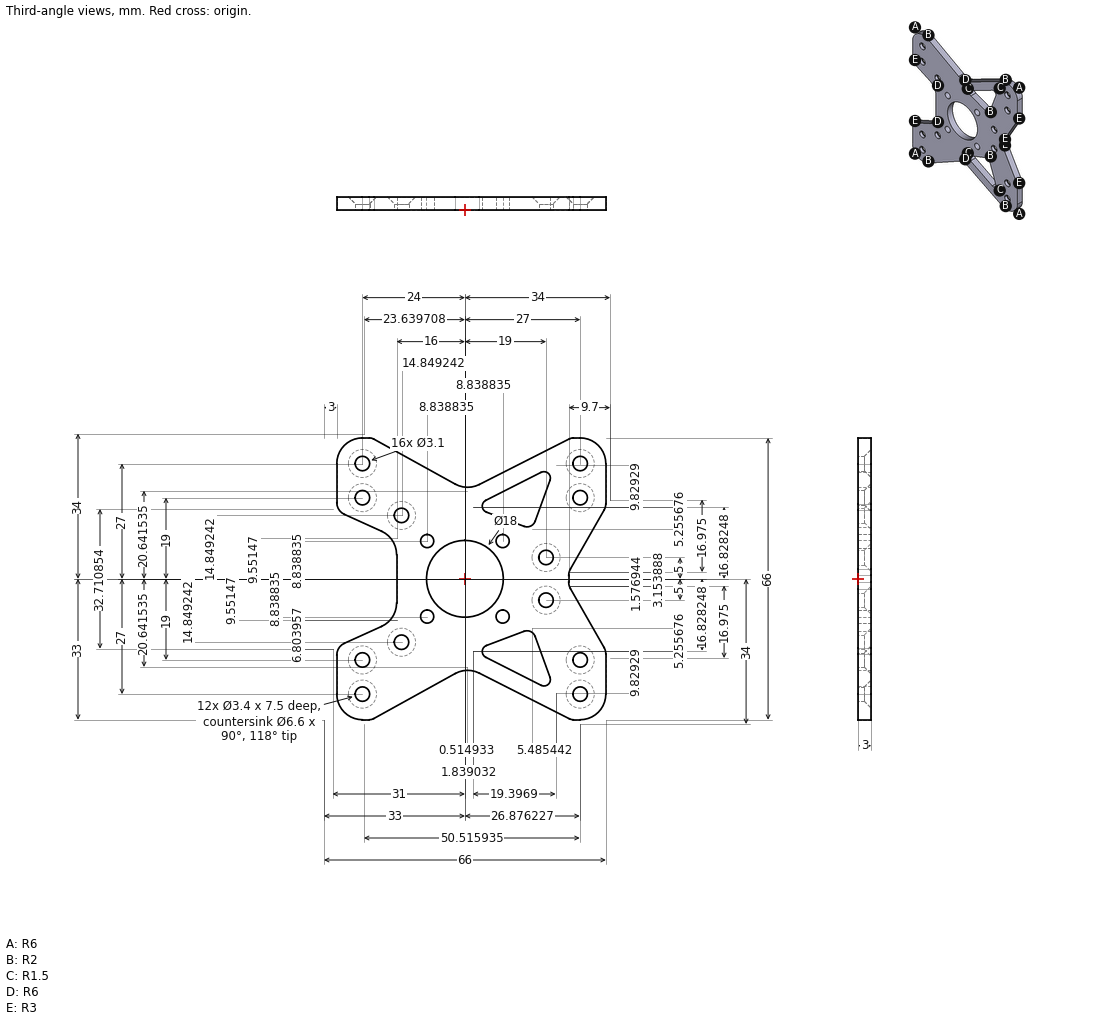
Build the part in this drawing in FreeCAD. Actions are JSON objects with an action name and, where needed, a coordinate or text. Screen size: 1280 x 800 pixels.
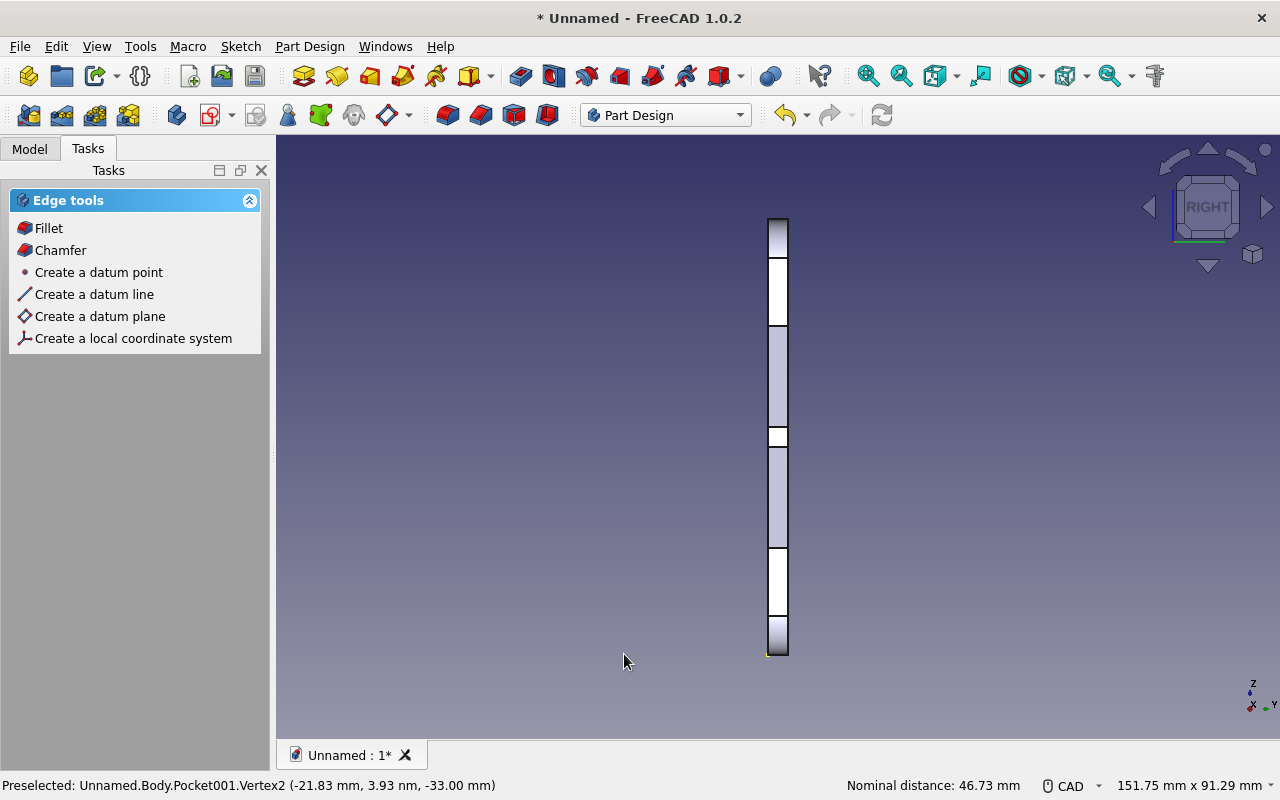
{"action": "scroll", "coordinate": [778, 654], "scroll_direction": "up", "scroll_amount": 4}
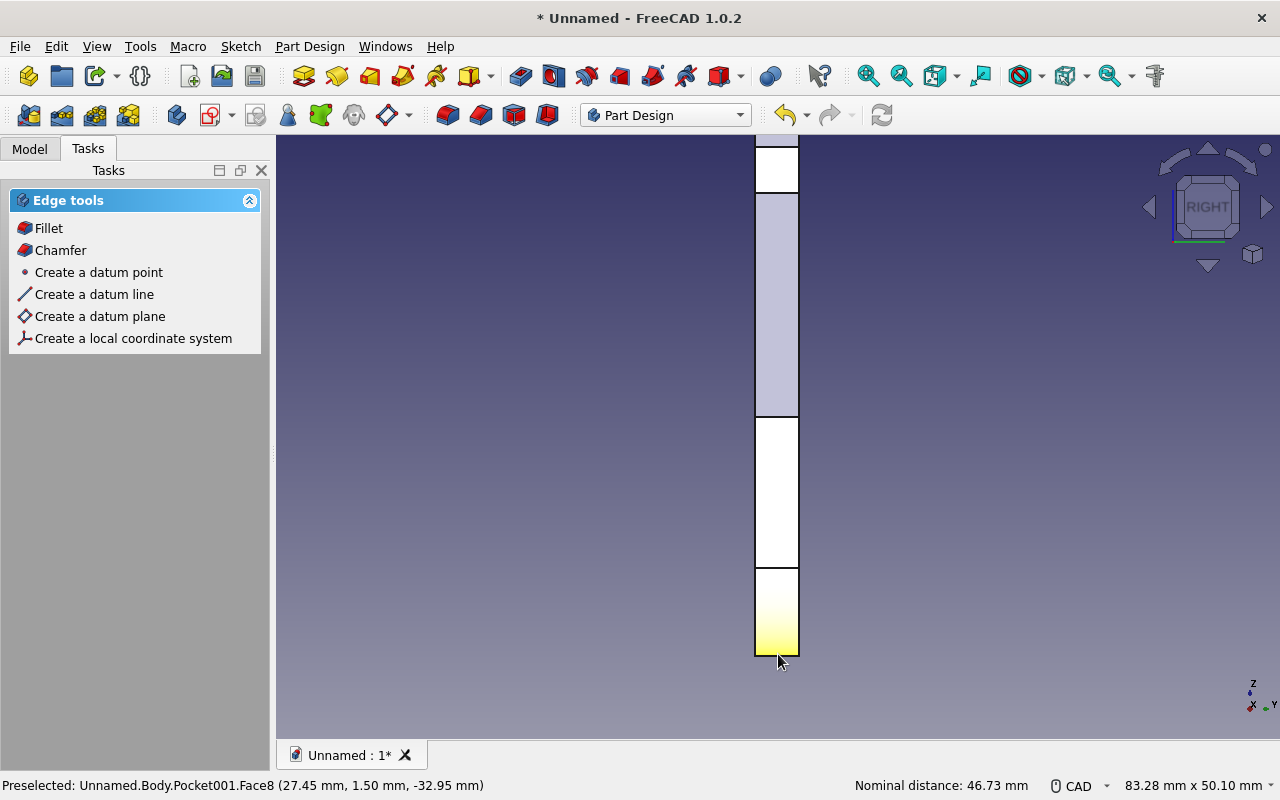
{"action": "key", "text": "v f"}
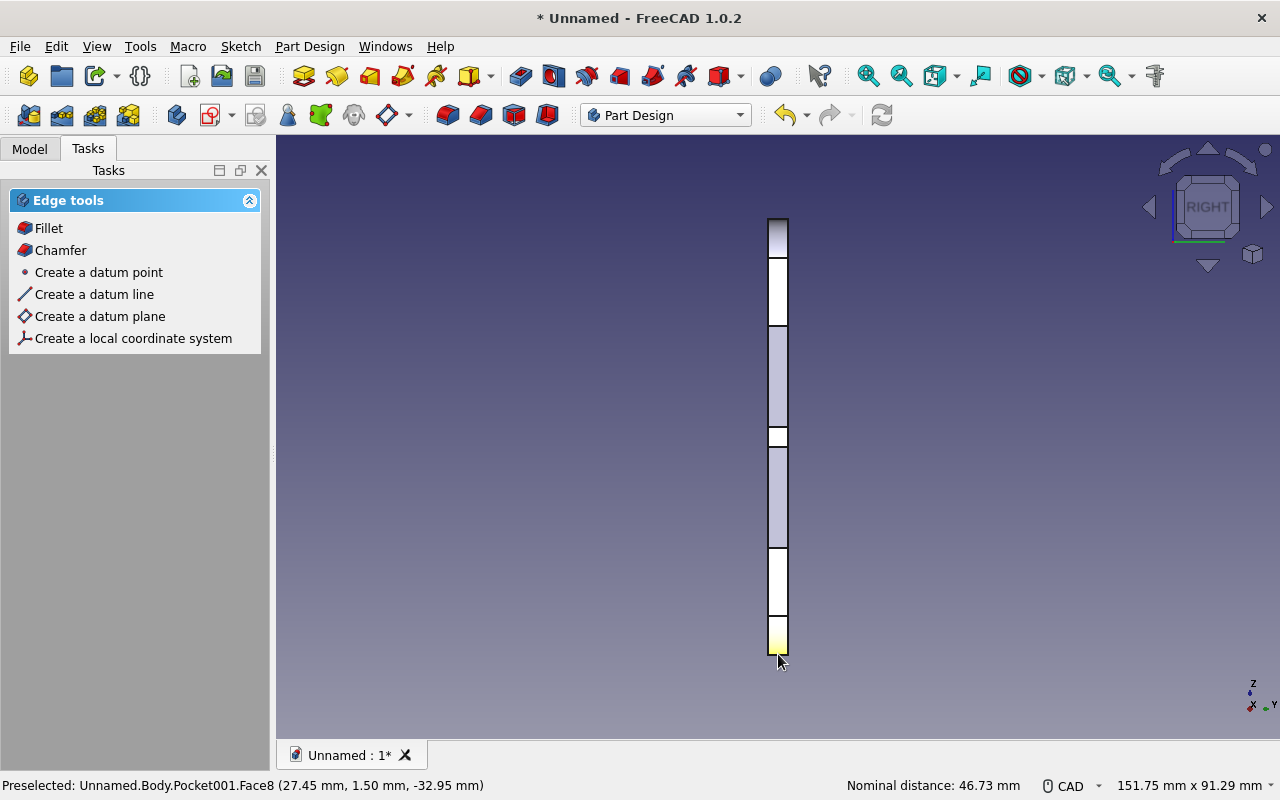
{"action": "key", "text": "5"}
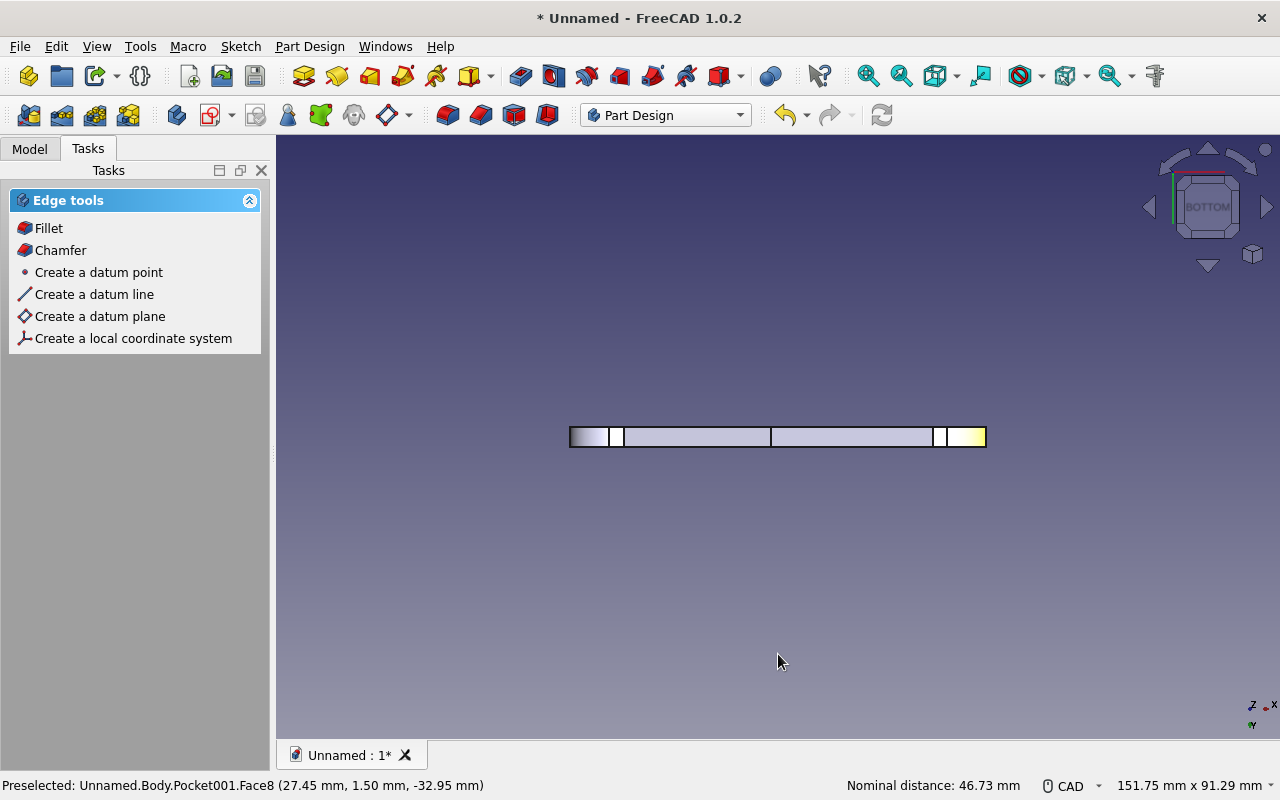
{"action": "key", "text": "v f"}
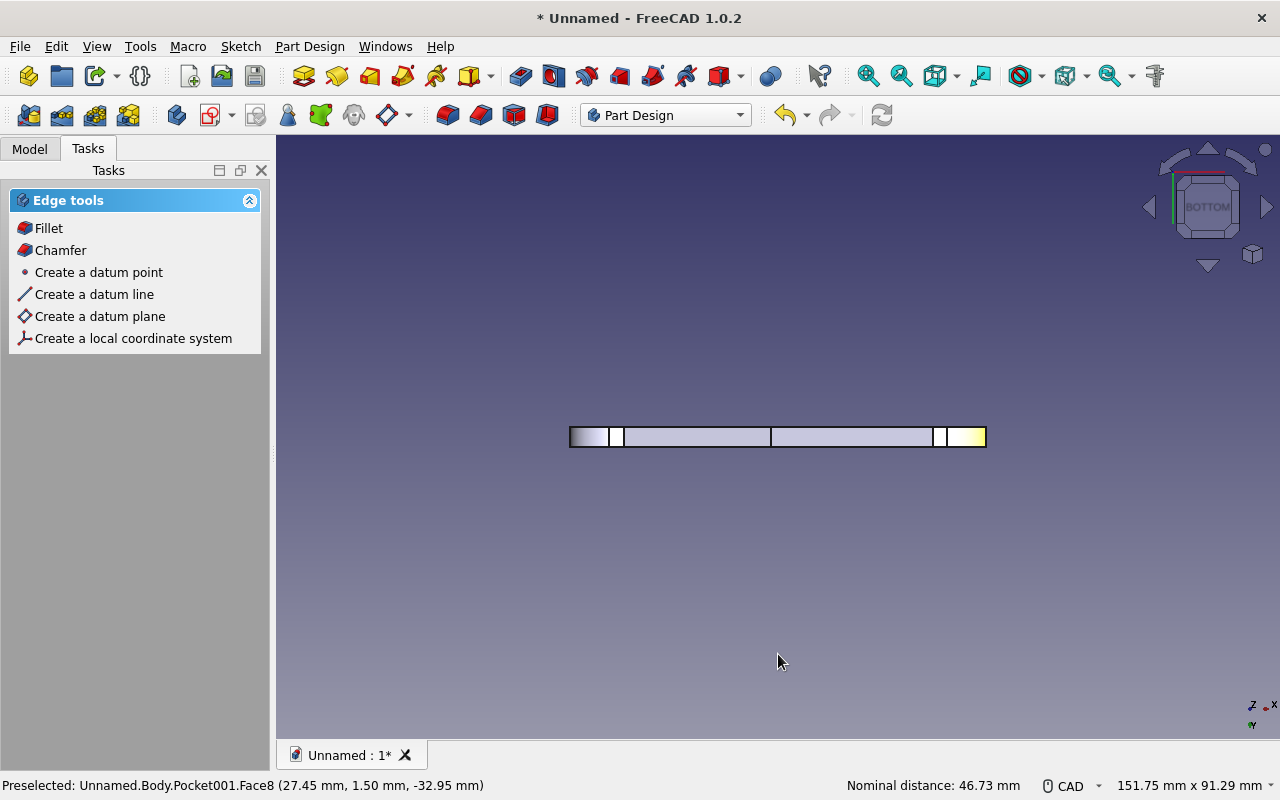
{"action": "left_click", "coordinate": [624, 436], "text": "ctrl"}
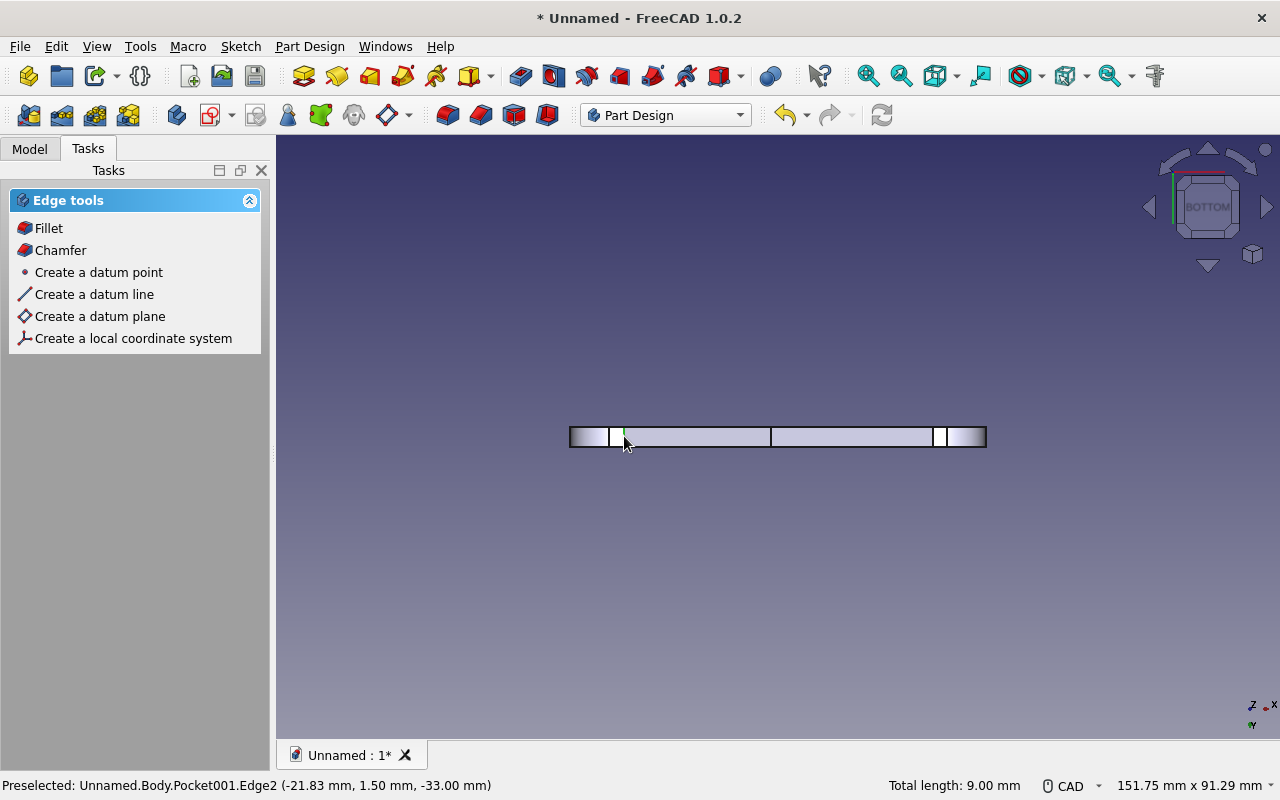
{"action": "left_click", "coordinate": [933, 436], "text": "ctrl"}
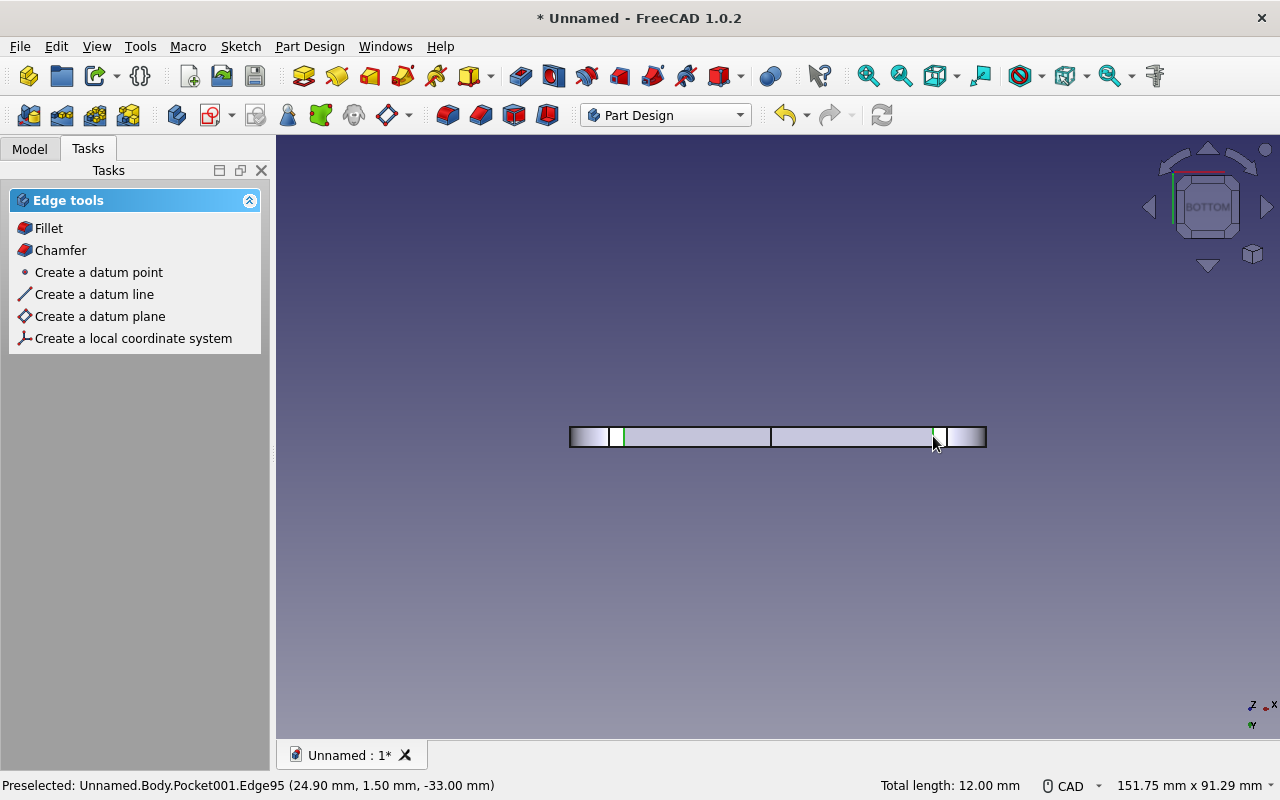
{"action": "scroll", "coordinate": [872, 436], "scroll_direction": "up", "scroll_amount": 4}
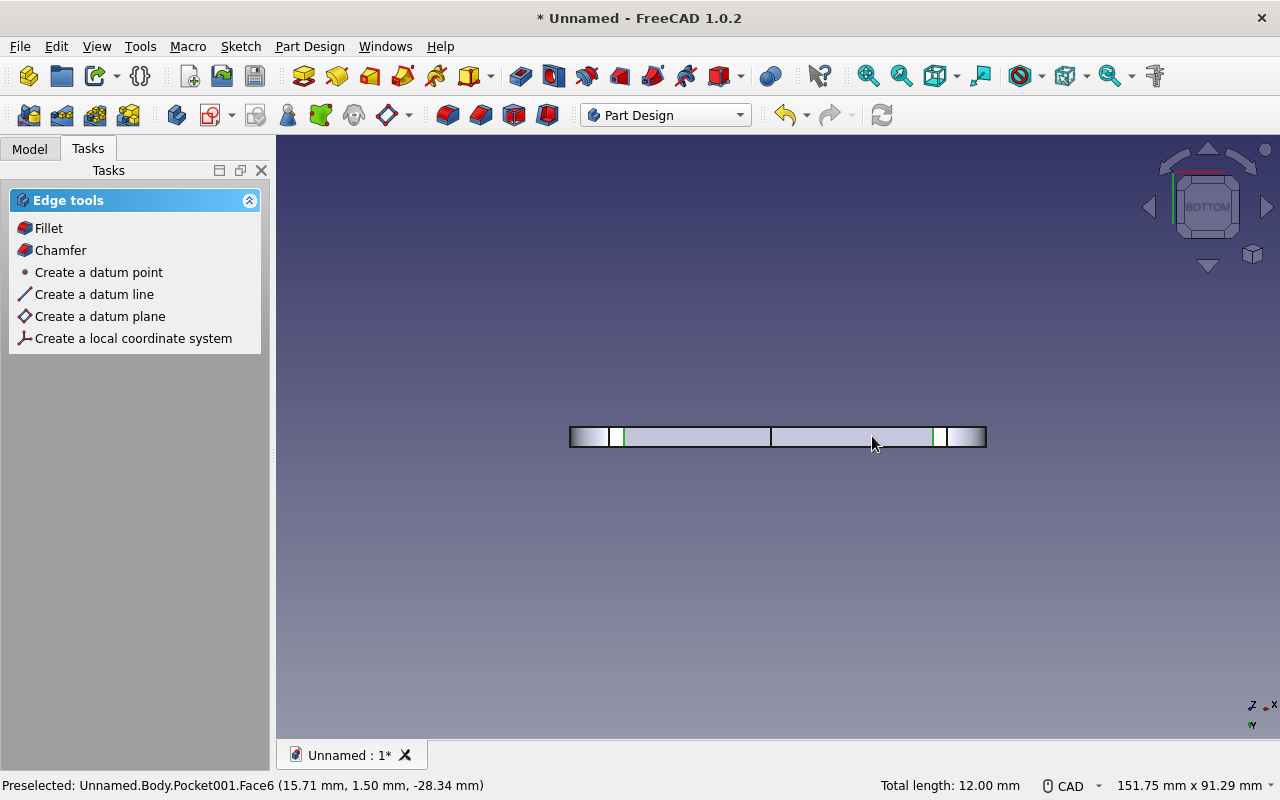
{"action": "left_click", "coordinate": [869, 76]}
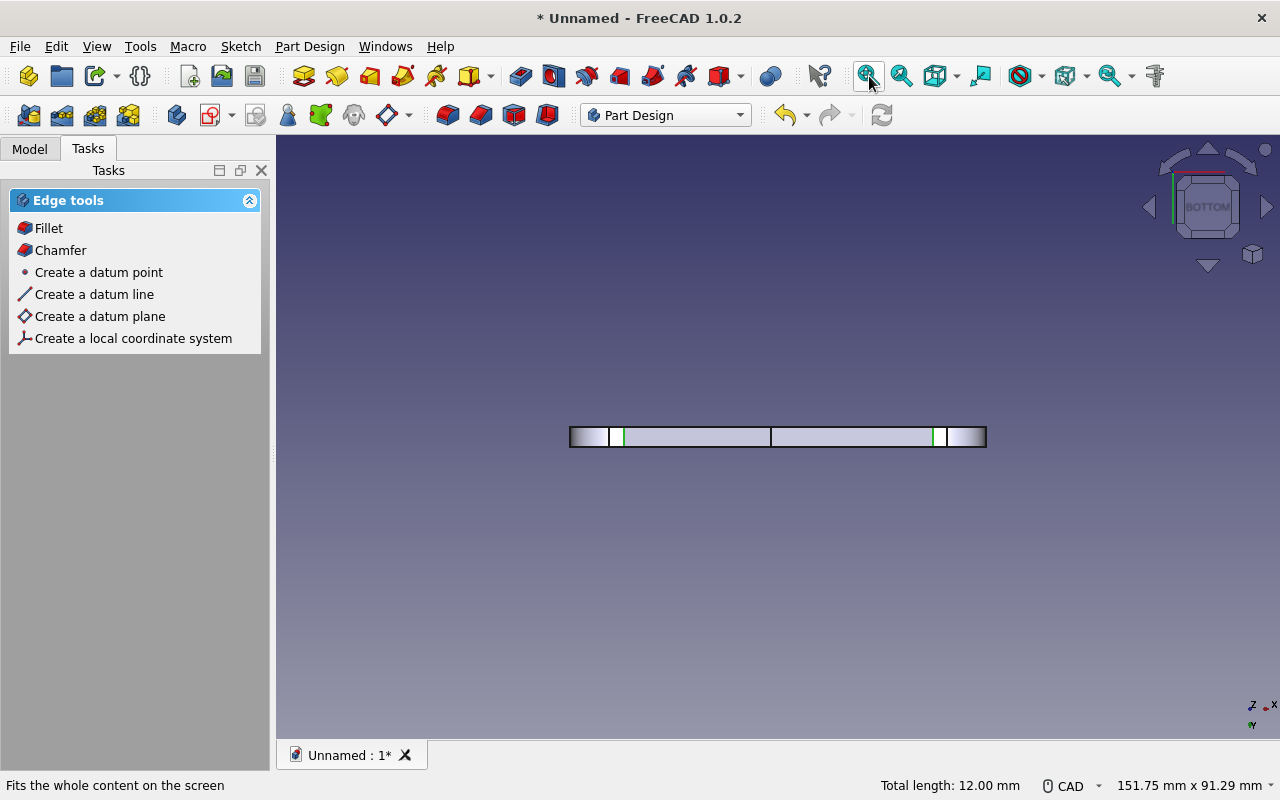
{"action": "key", "text": "4"}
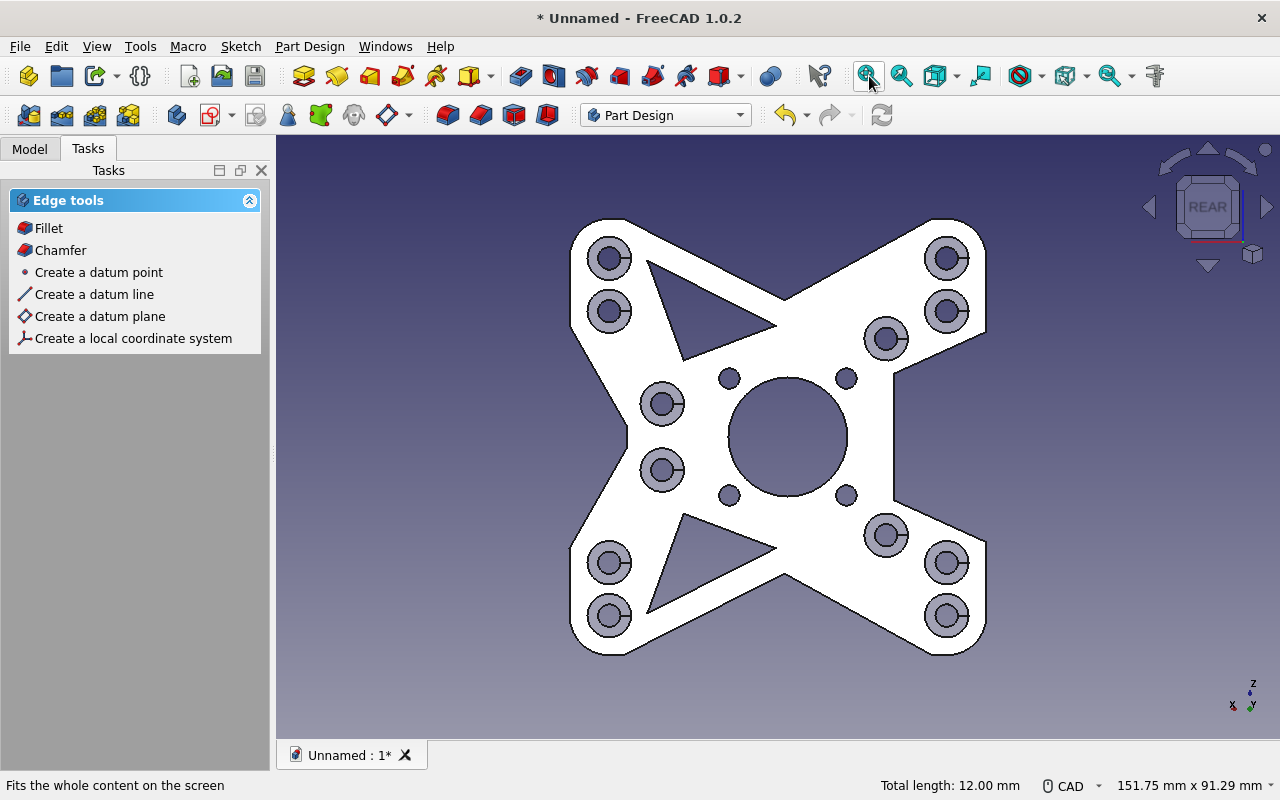
{"action": "scroll", "coordinate": [684, 359], "scroll_direction": "up", "scroll_amount": 4}